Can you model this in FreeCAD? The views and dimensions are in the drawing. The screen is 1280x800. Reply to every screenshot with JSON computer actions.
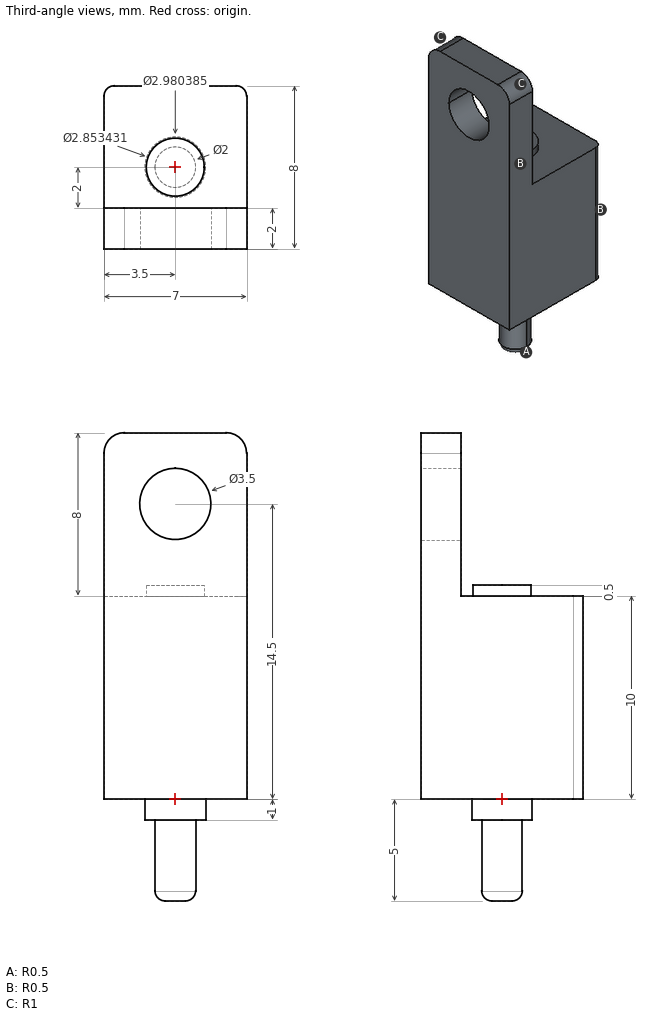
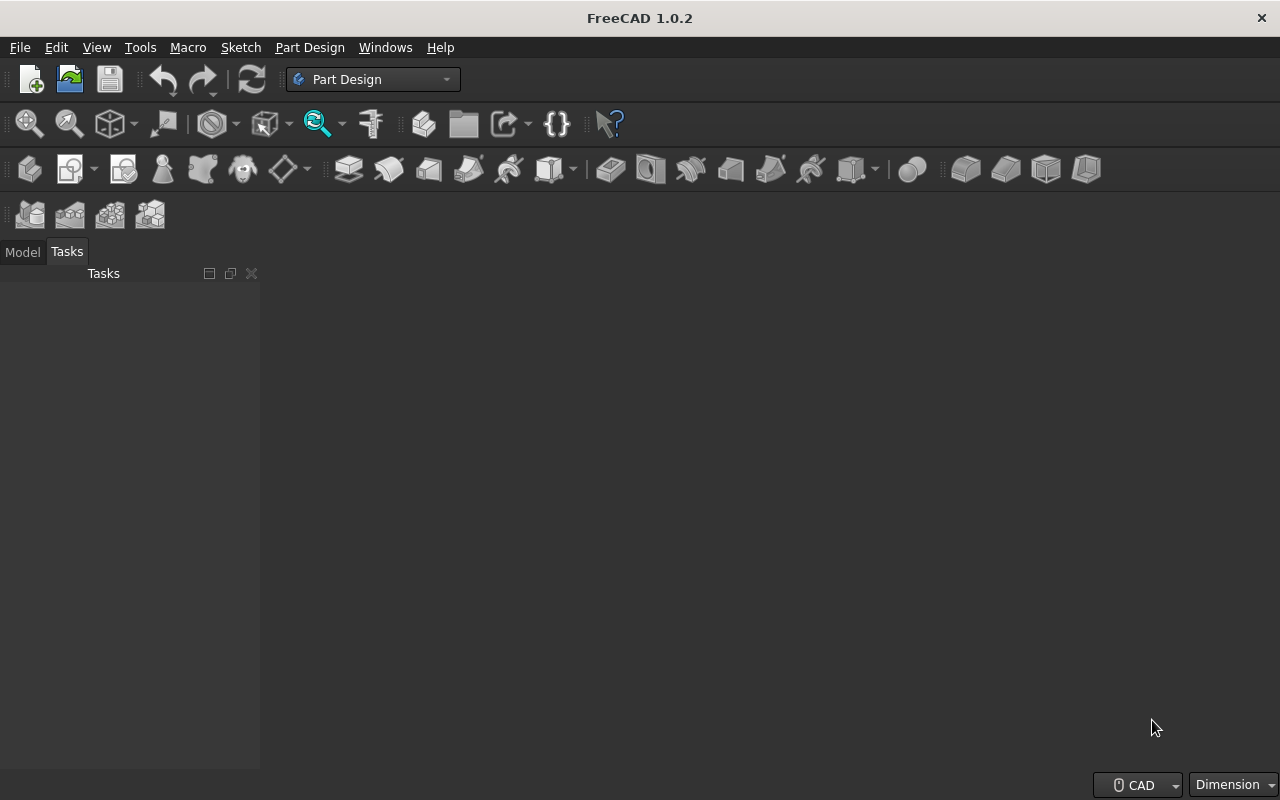
{"action": "key", "text": "ctrl+n"}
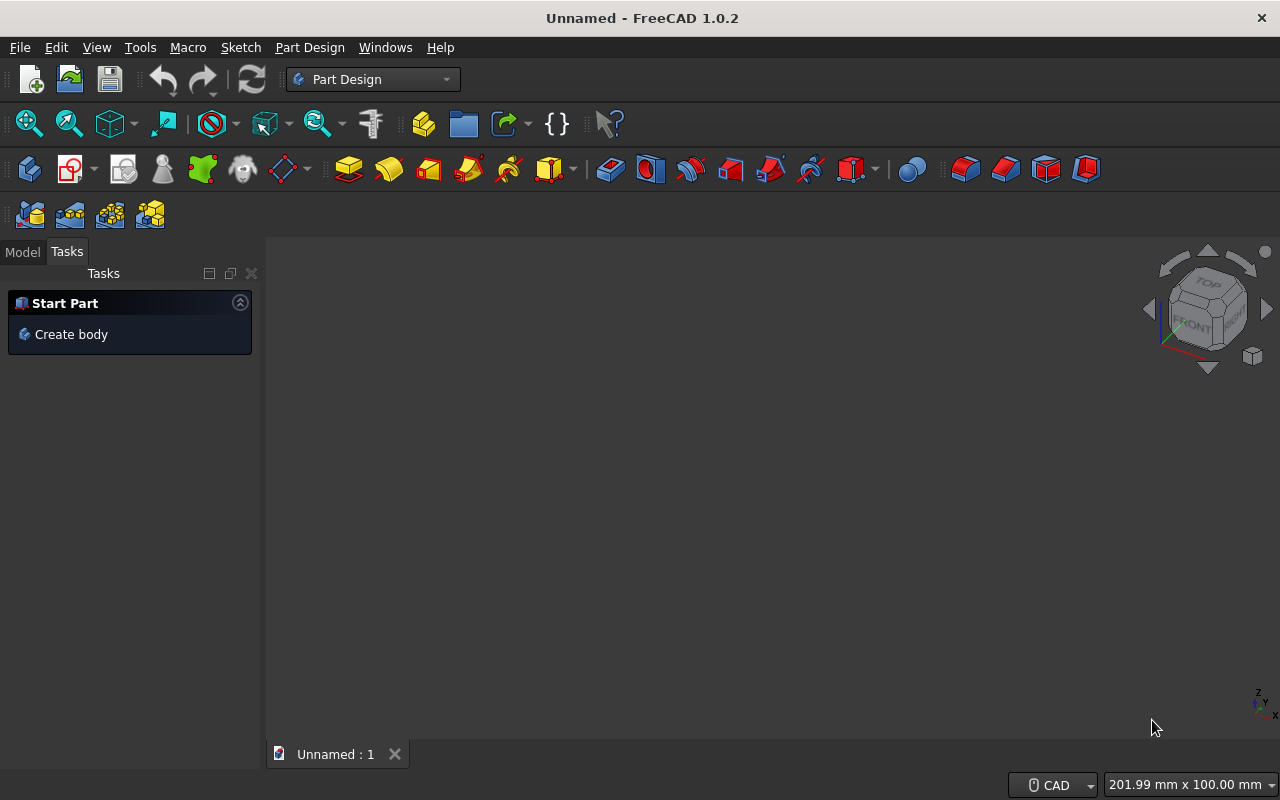
{"action": "left_click", "coordinate": [70, 170]}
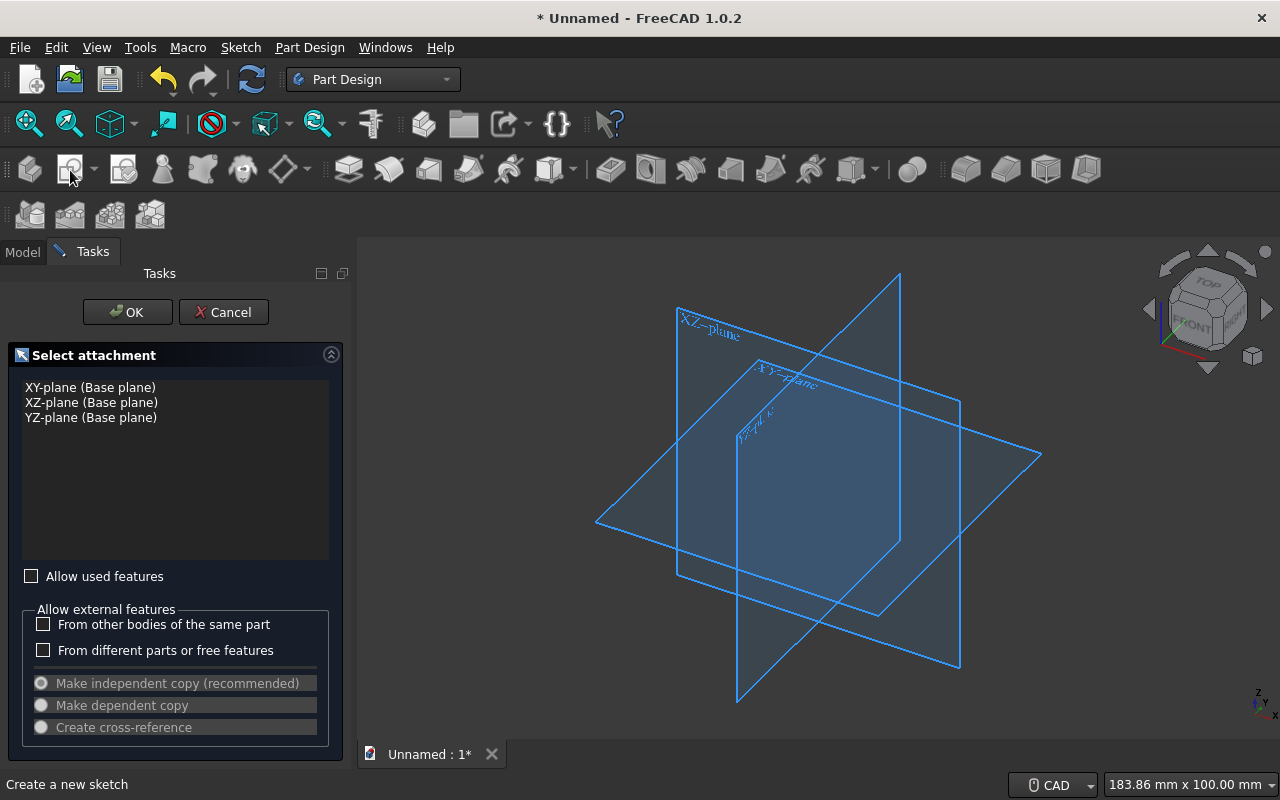
{"action": "left_click", "coordinate": [82, 388]}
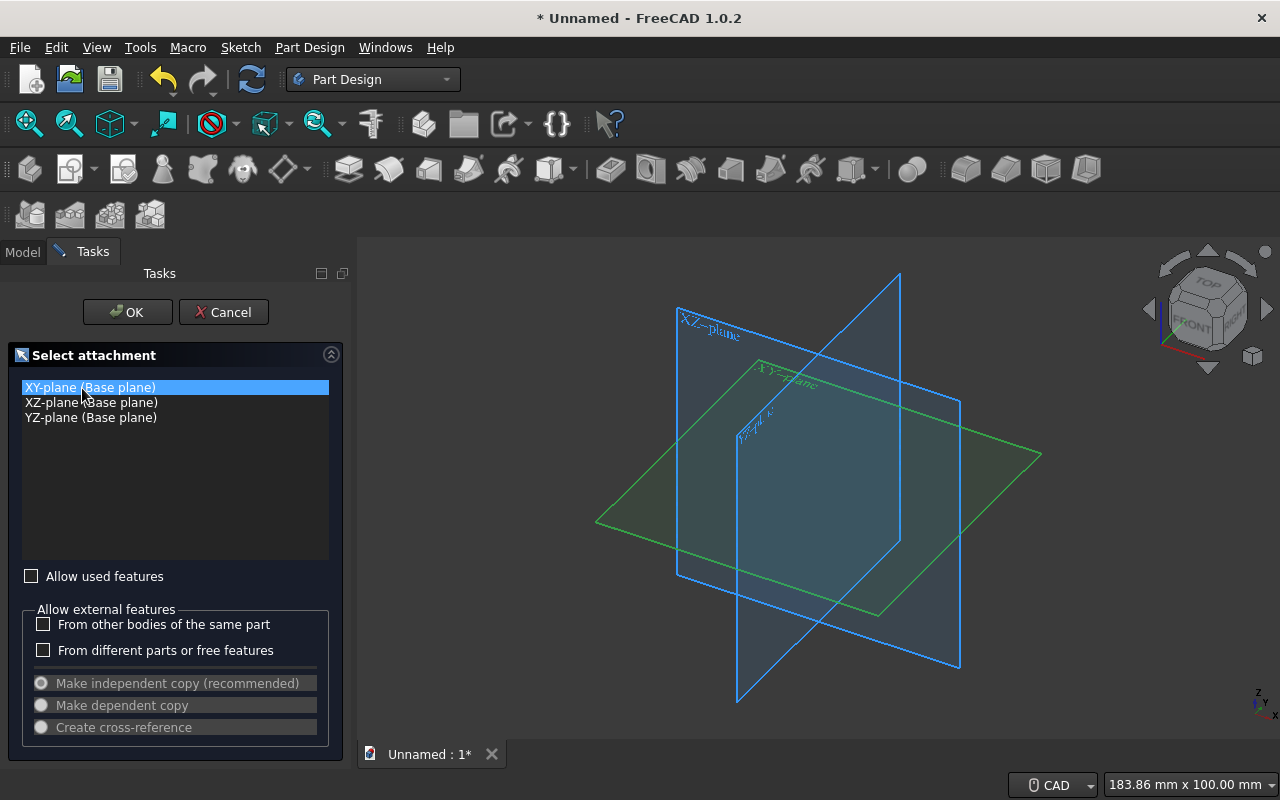
{"action": "left_click", "coordinate": [128, 312]}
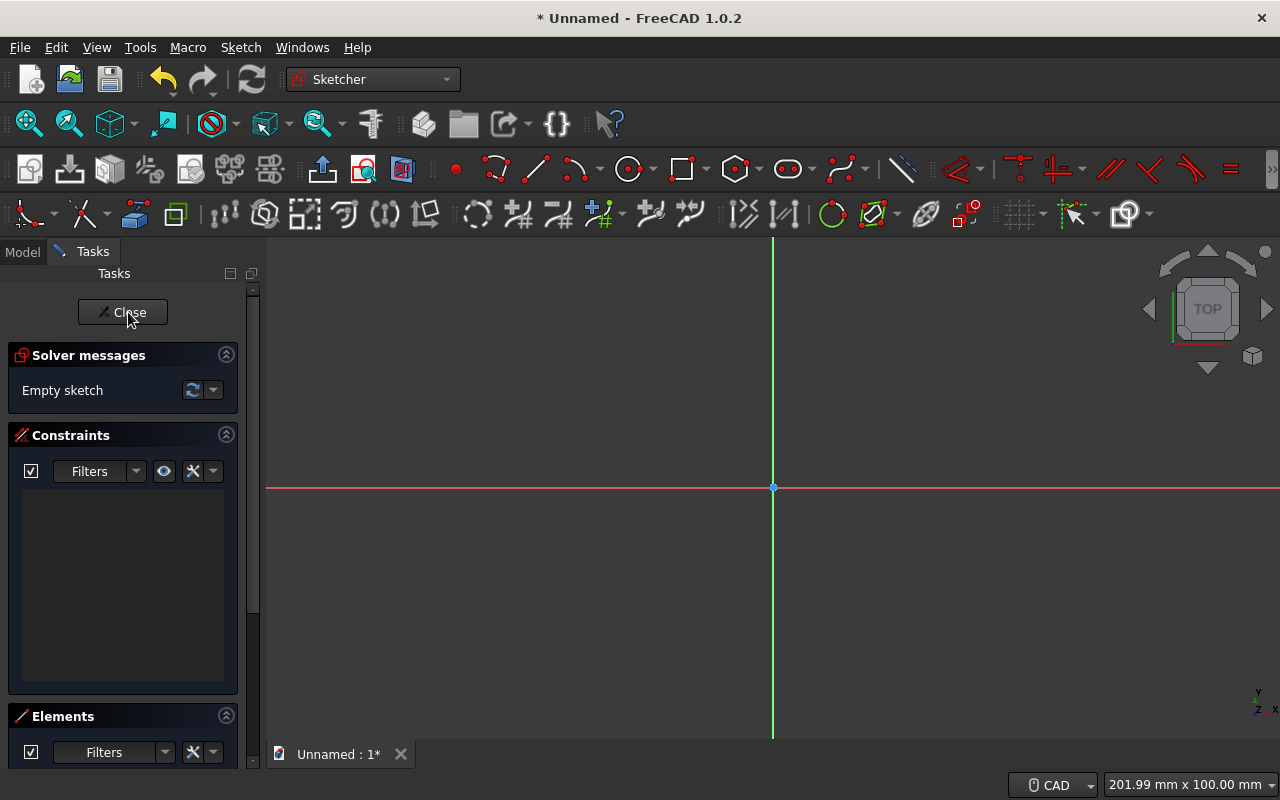
{"action": "scroll", "coordinate": [784, 488], "scroll_direction": "up", "scroll_amount": 10}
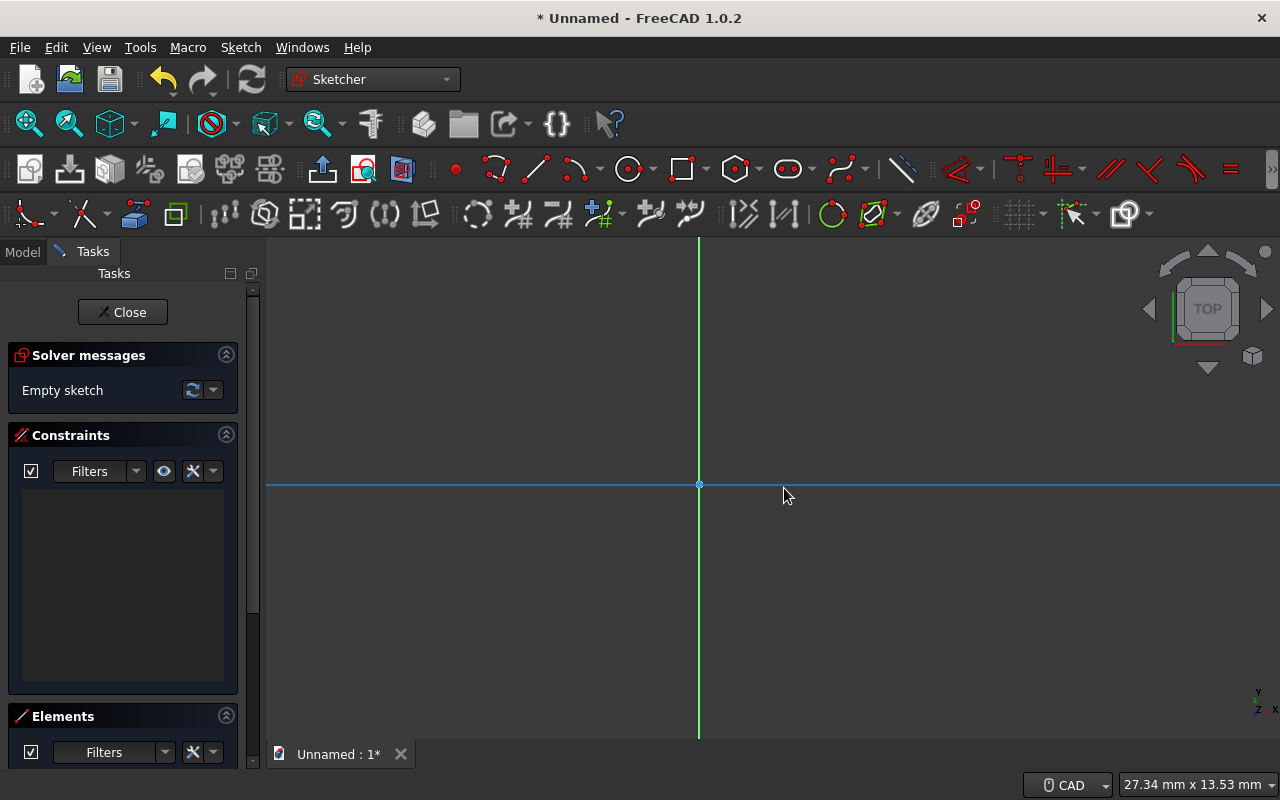
{"action": "key", "text": "g v"}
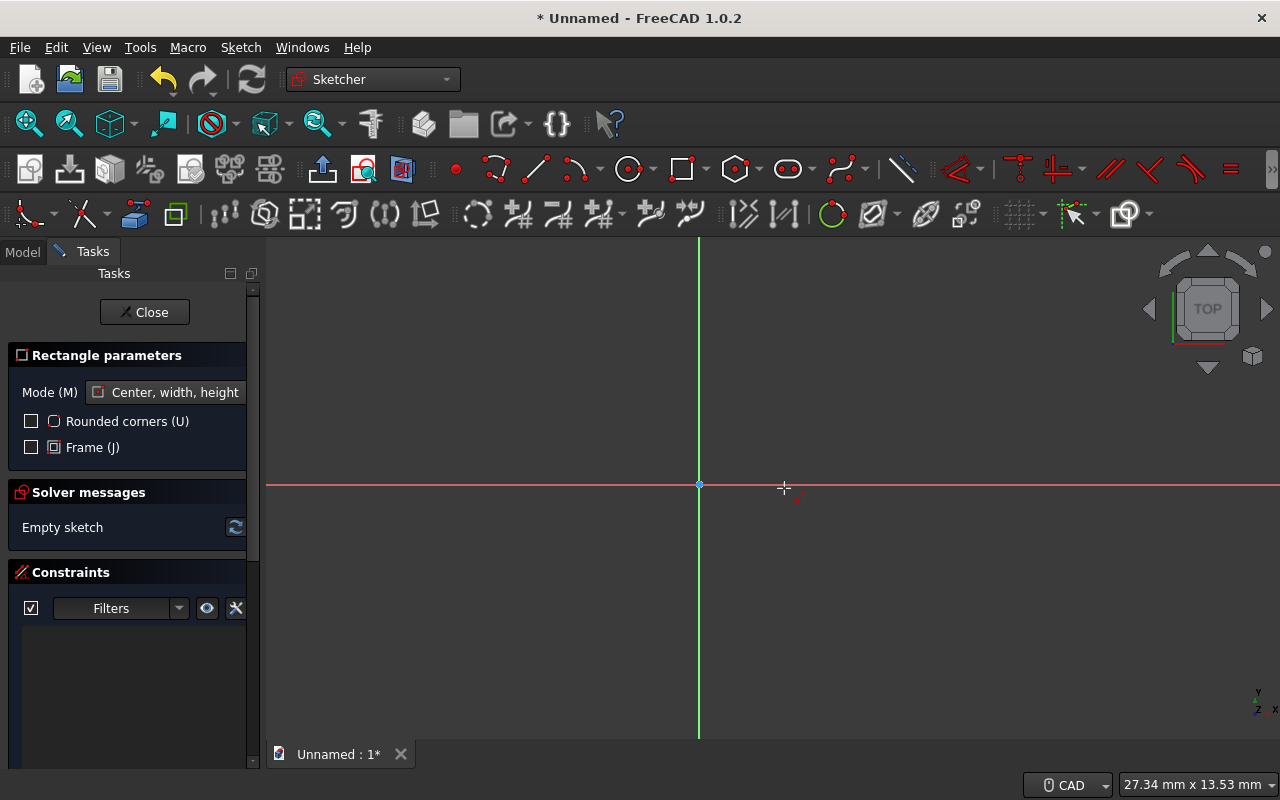
{"action": "left_click", "coordinate": [699, 485]}
{"action": "mouse_move", "coordinate": [829, 336]}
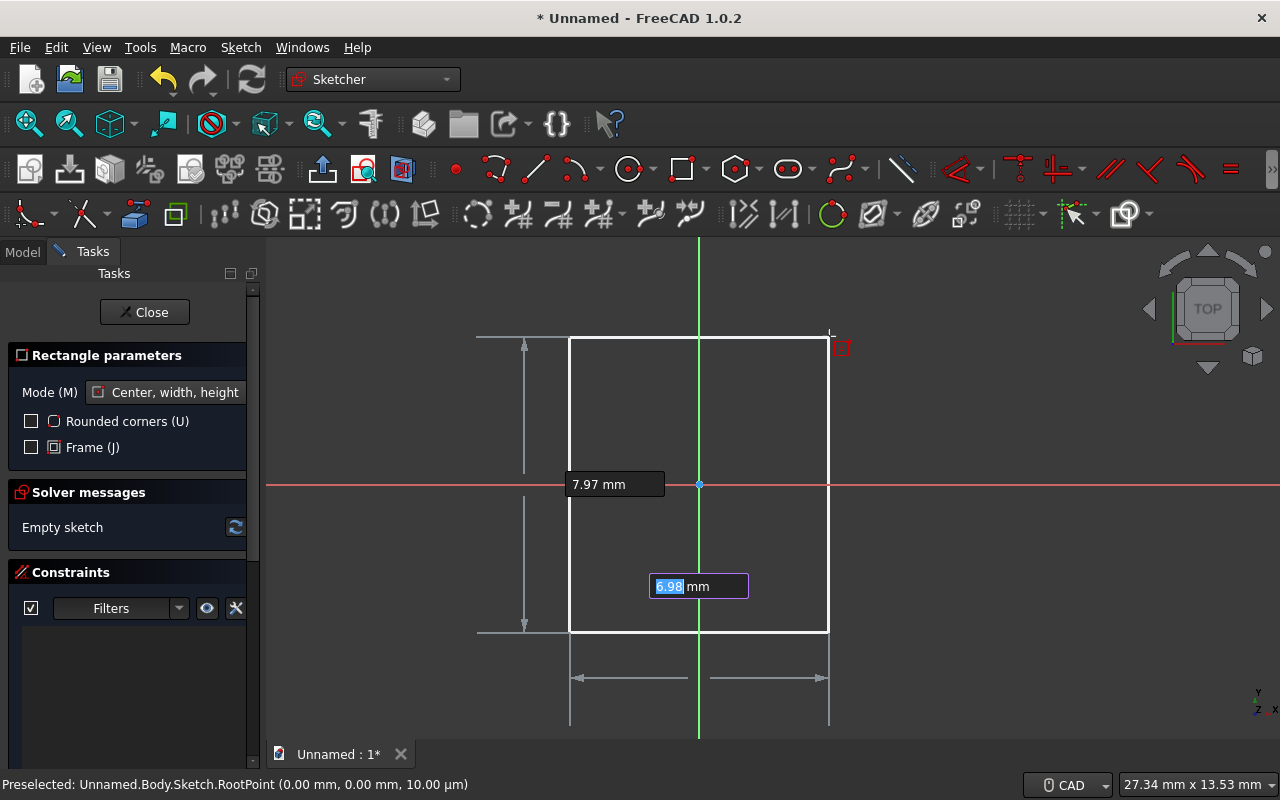
{"action": "type", "text": "7"}
{"action": "key", "text": "Tab"}
{"action": "type", "text": "8"}
{"action": "key", "text": "Return"}
{"action": "key", "text": "Escape"}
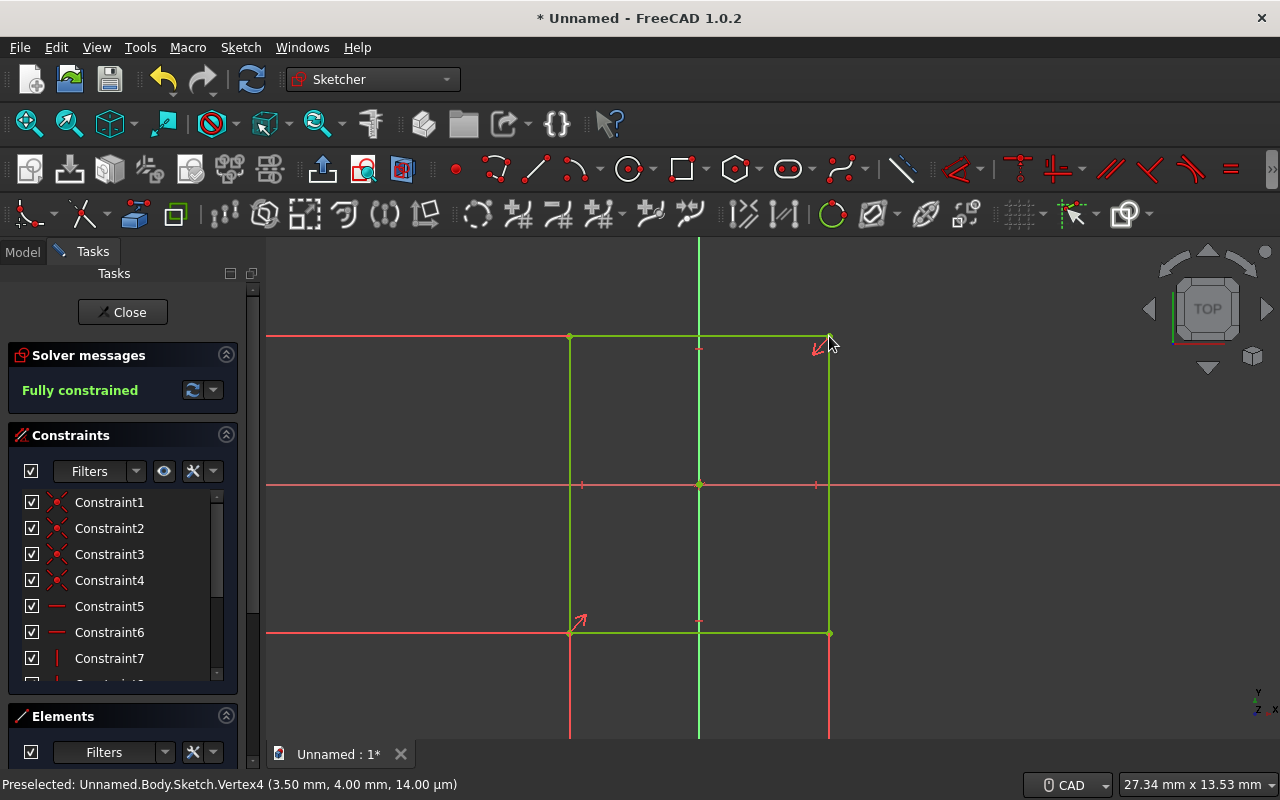
{"action": "left_click", "coordinate": [123, 312]}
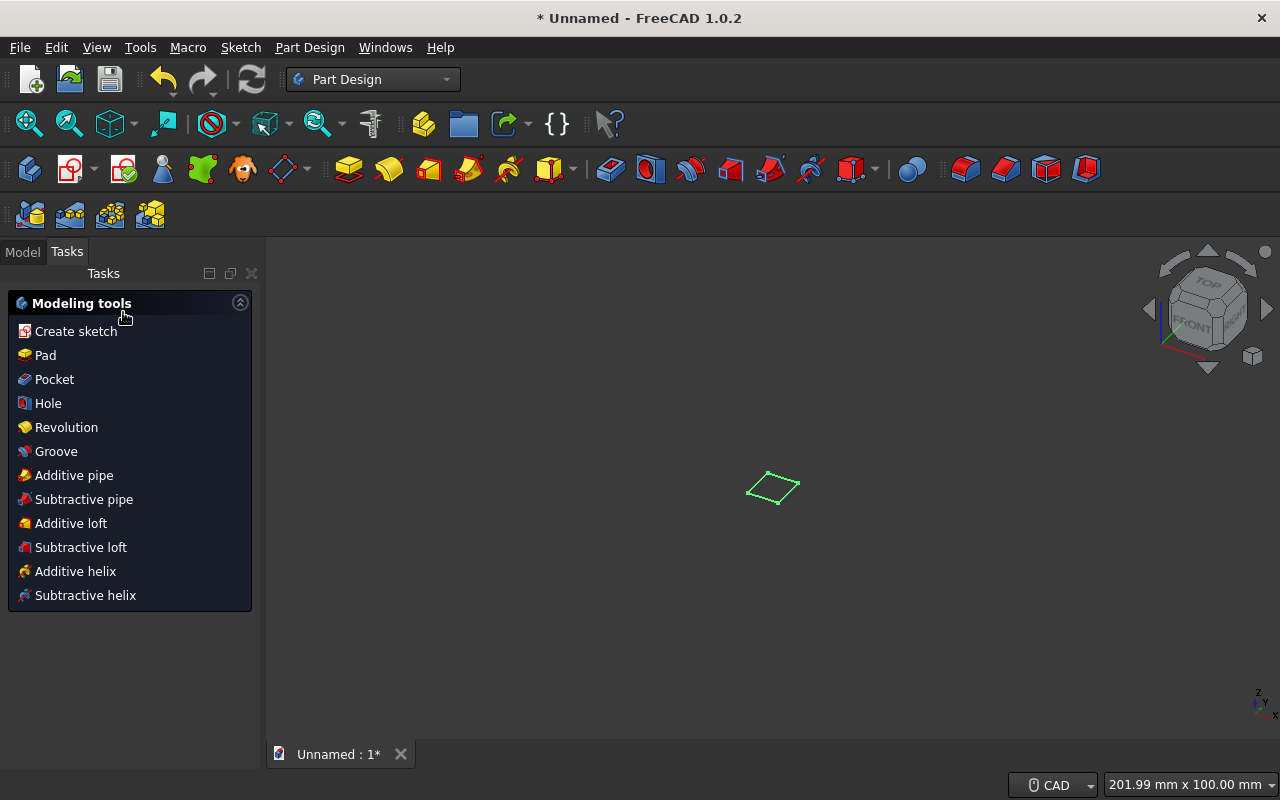
{"action": "left_click", "coordinate": [350, 170]}